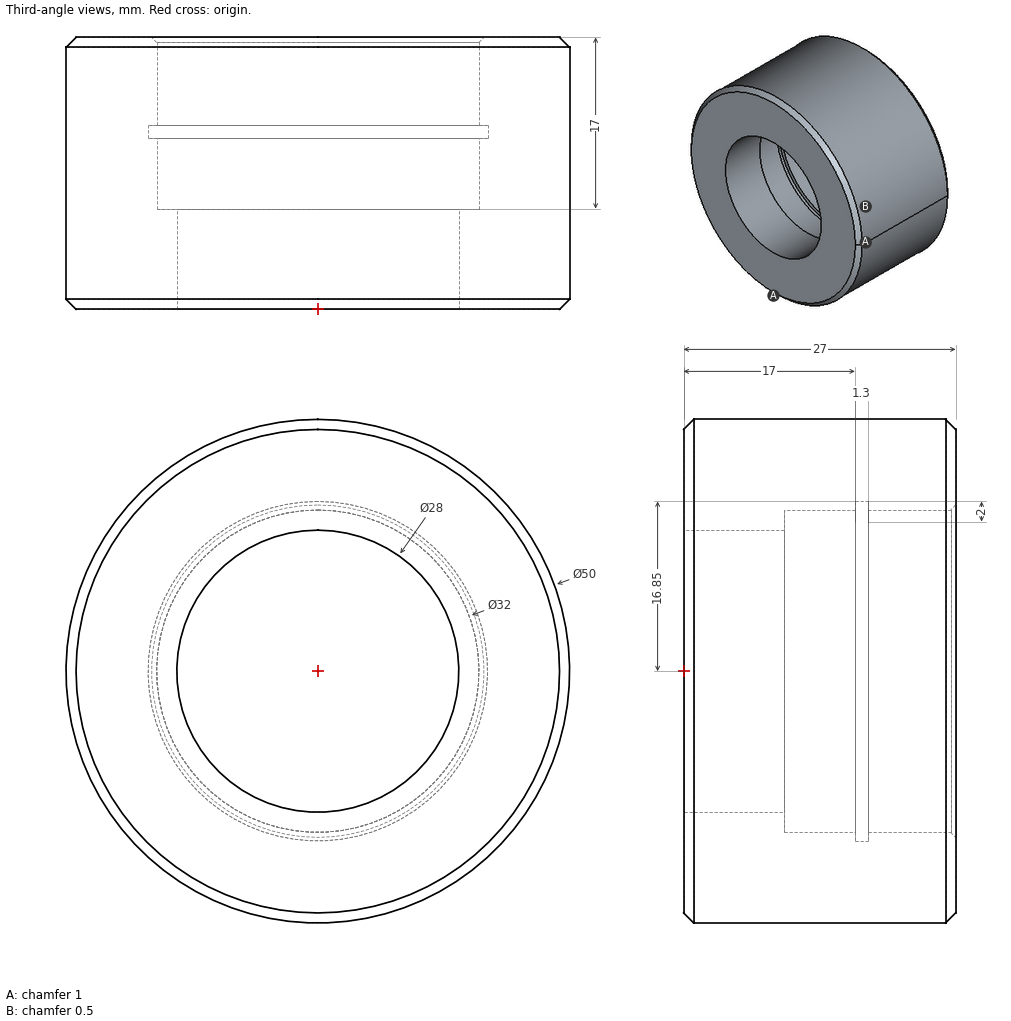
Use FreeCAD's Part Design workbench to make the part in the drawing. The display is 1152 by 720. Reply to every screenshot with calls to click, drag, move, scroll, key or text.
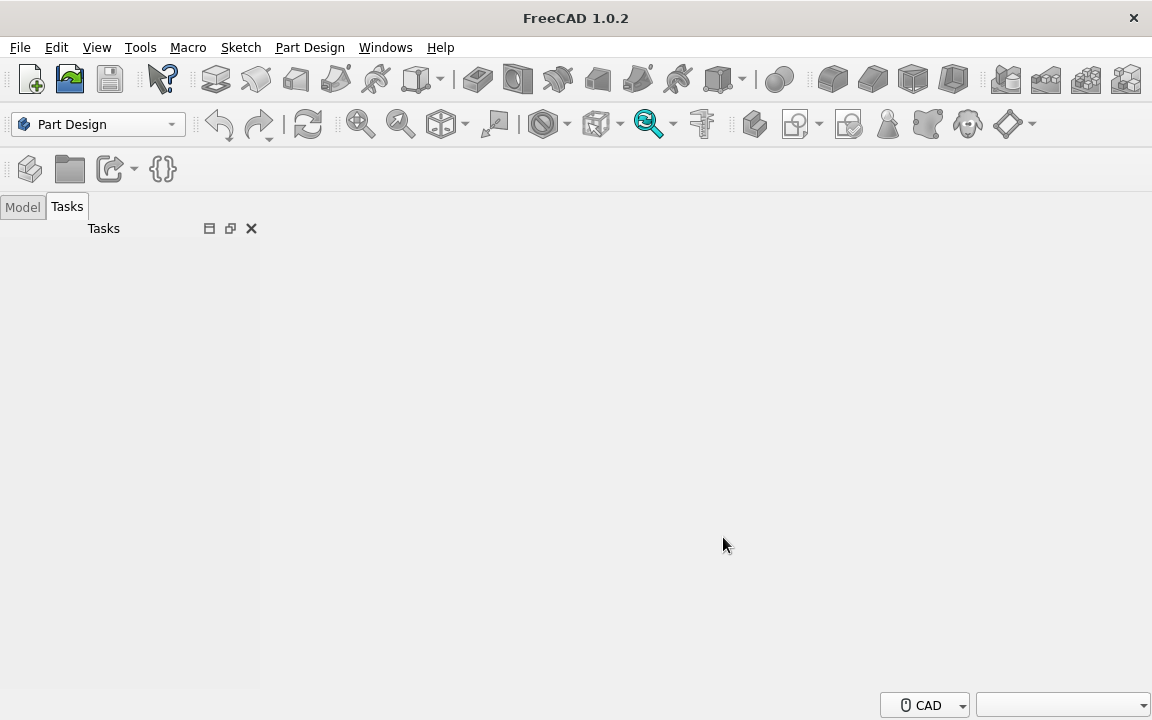
click(30, 80)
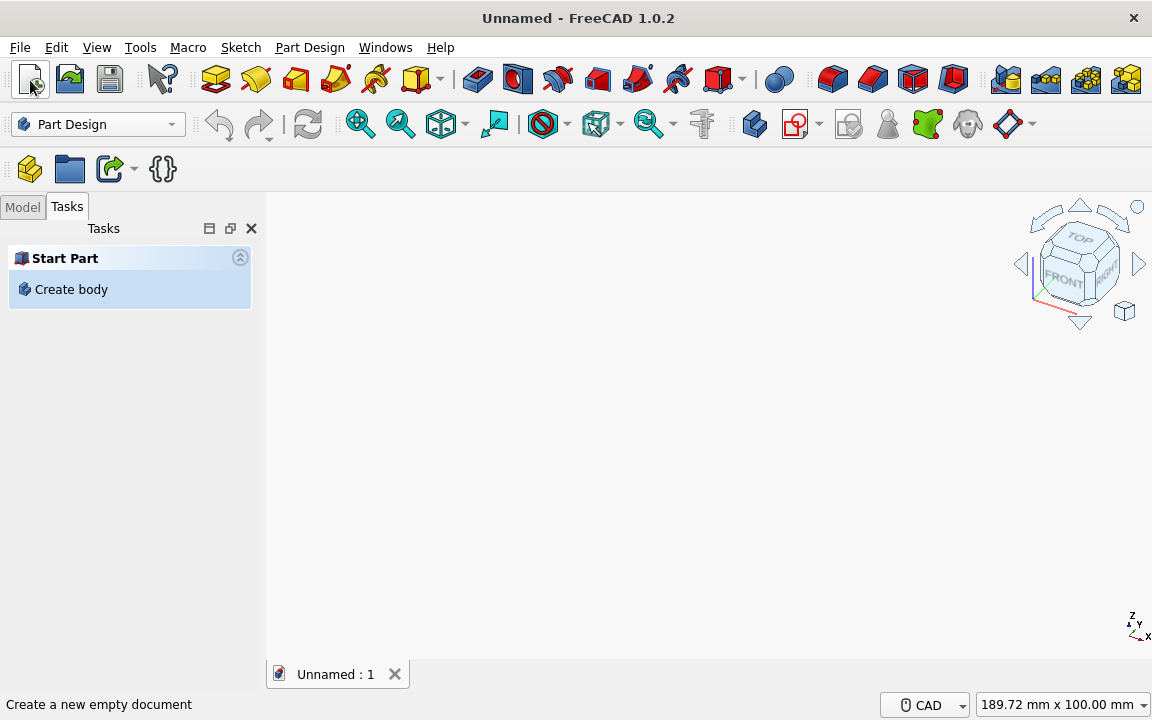
click(796, 124)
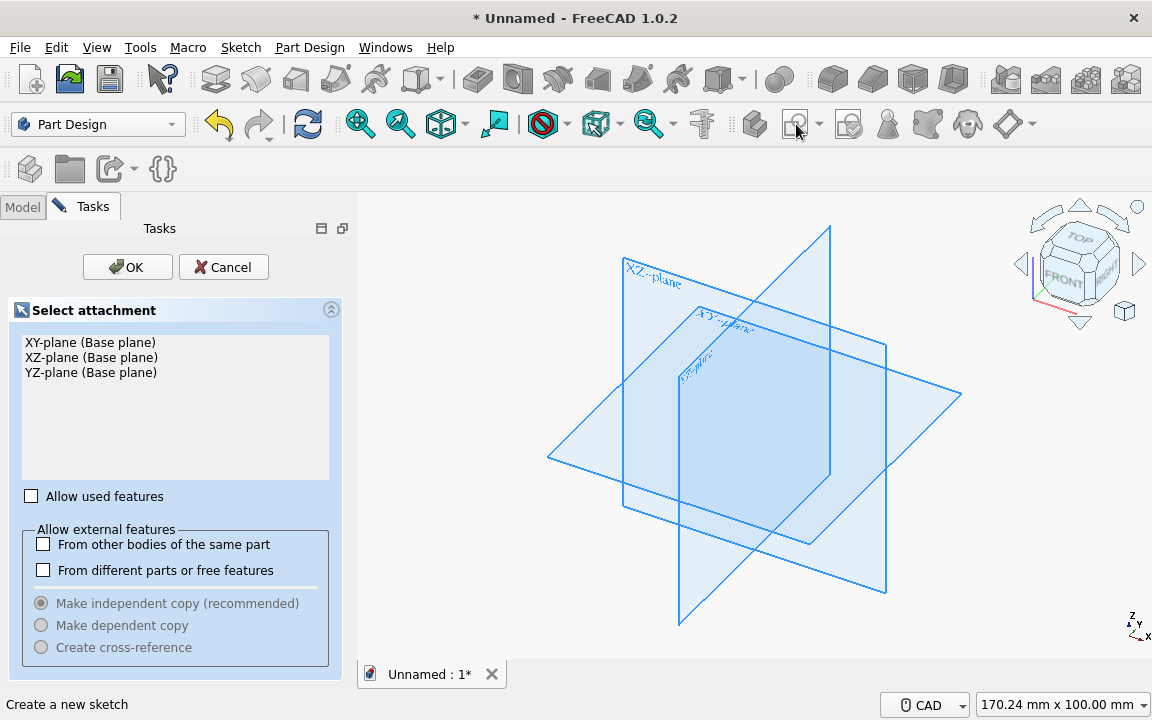
click(82, 358)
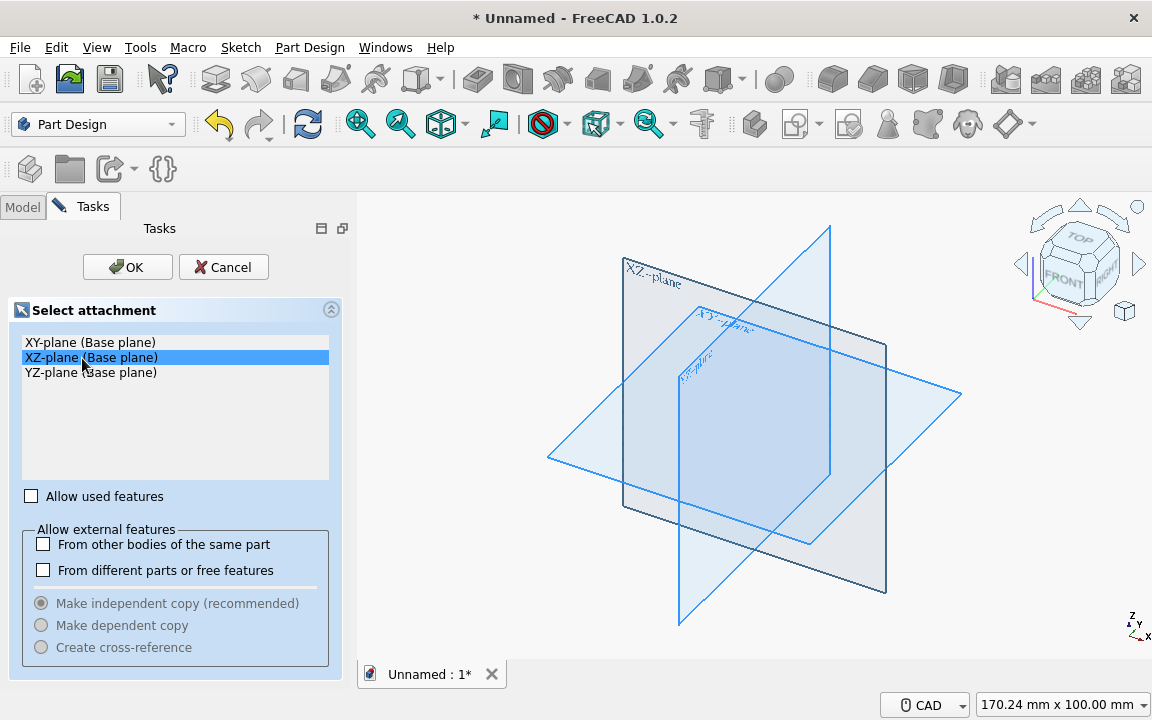
click(128, 267)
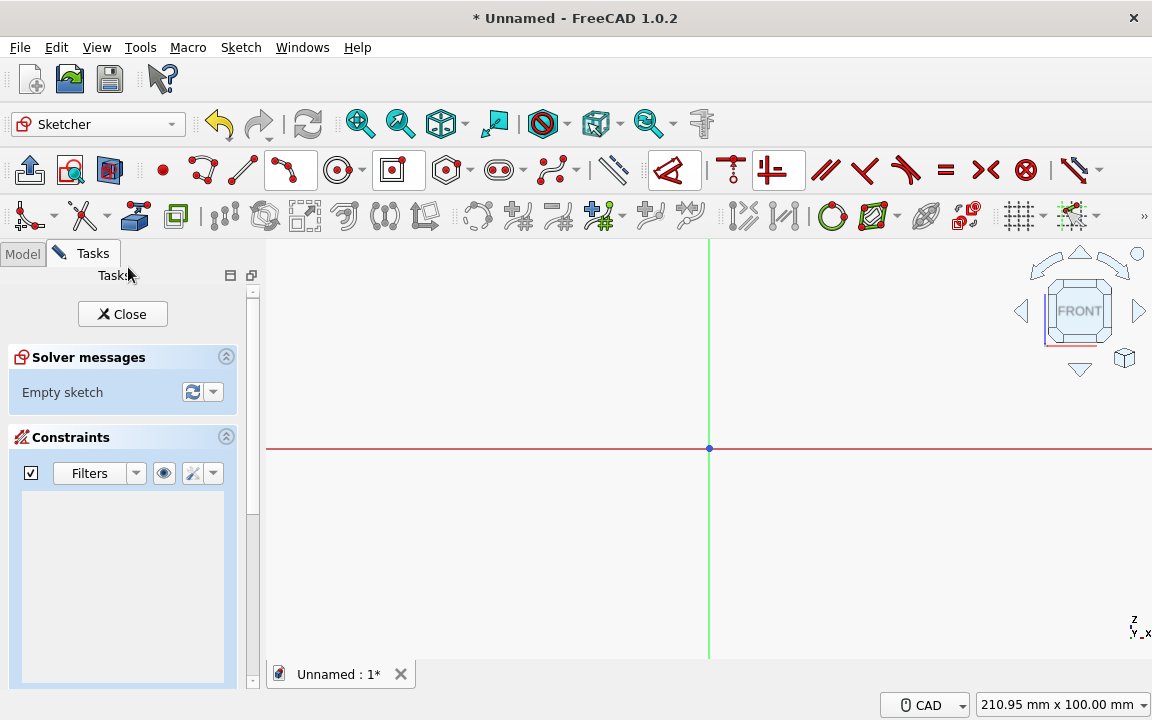
click(338, 170)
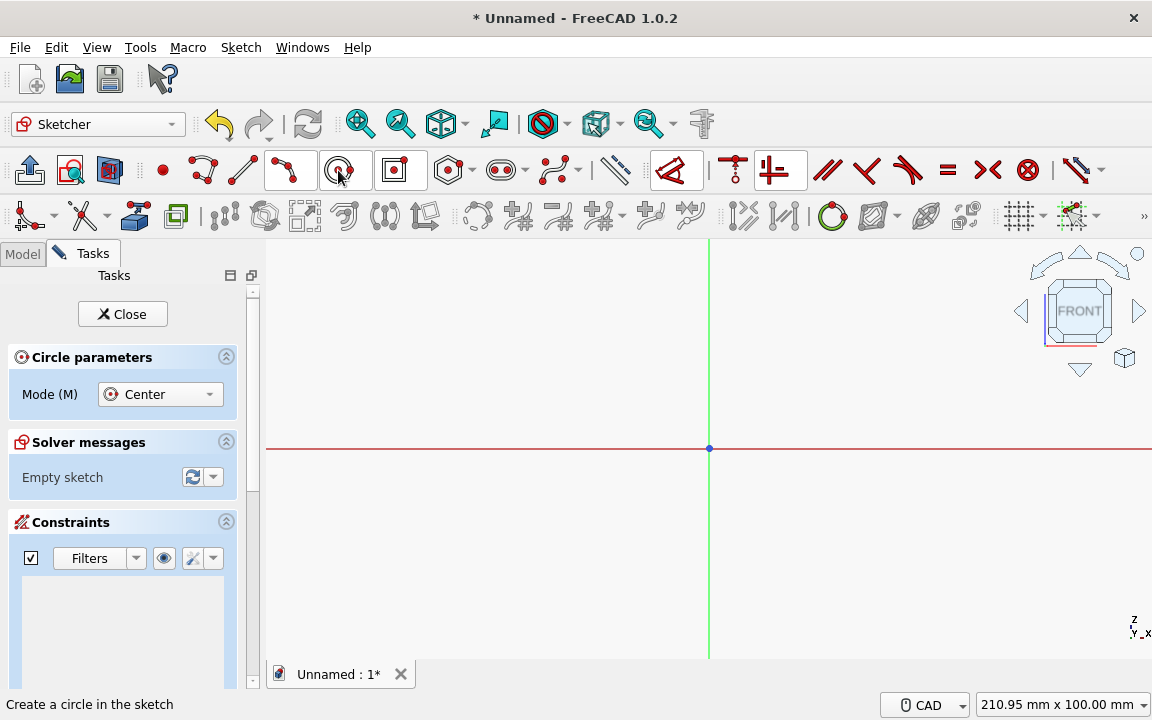
click(709, 449)
move(783, 375)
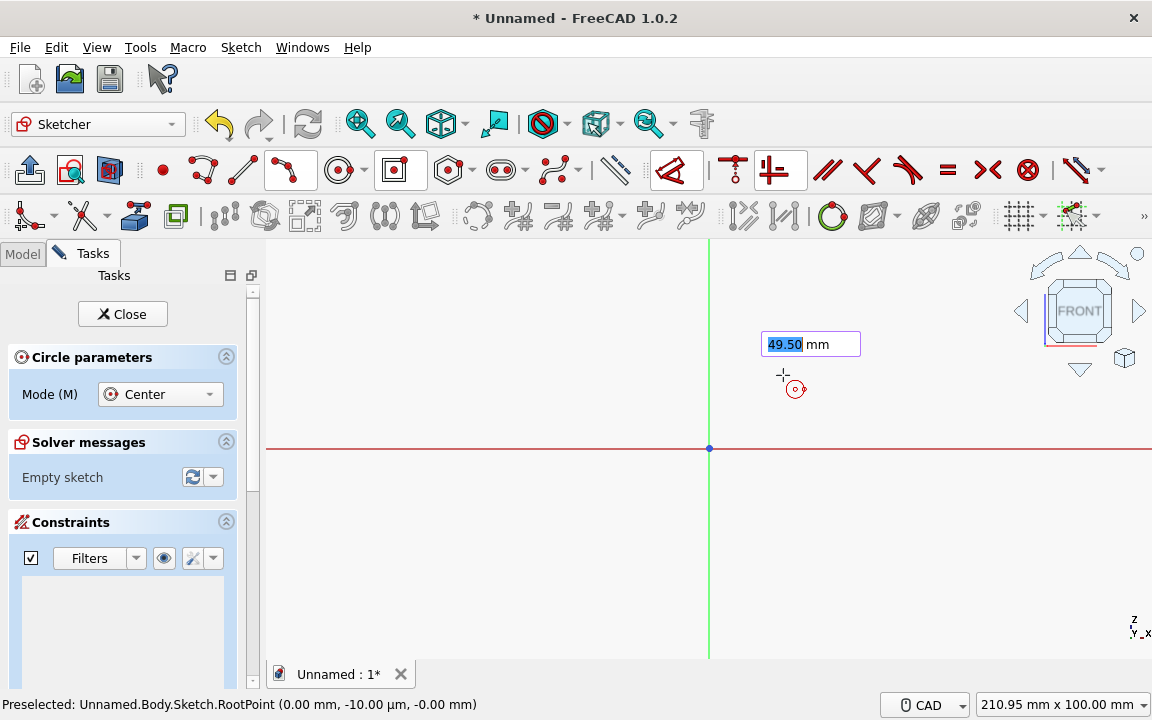
text(50)
key(Return)
key(Escape)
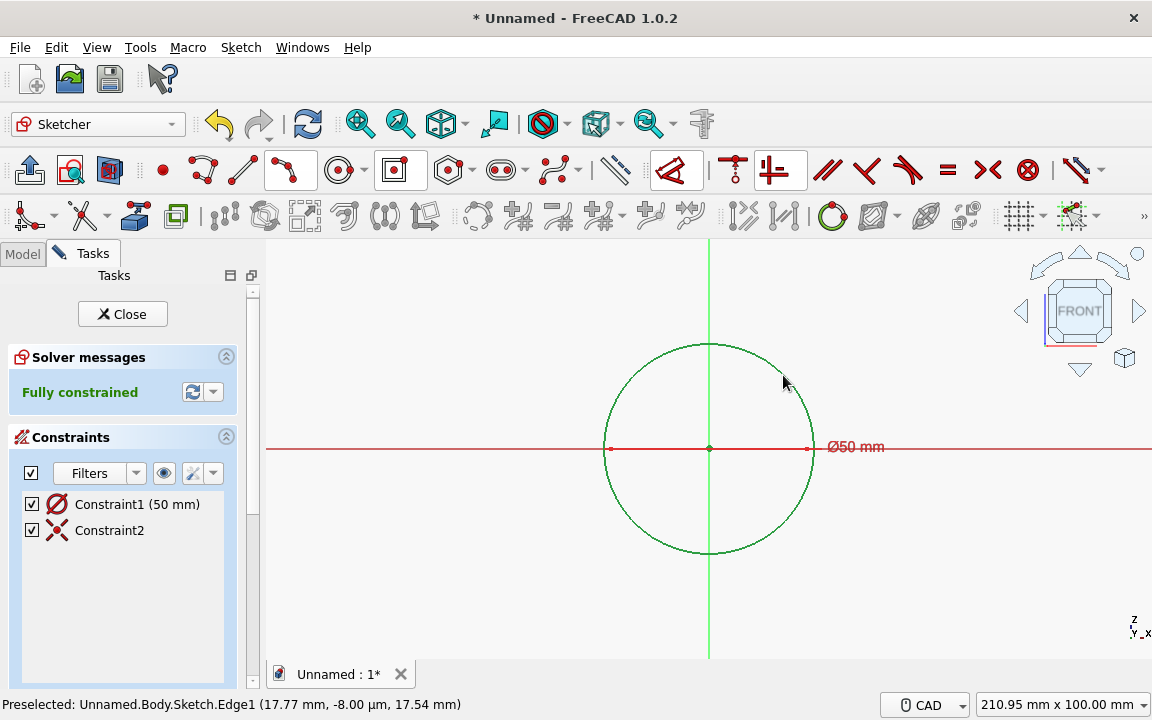
click(123, 314)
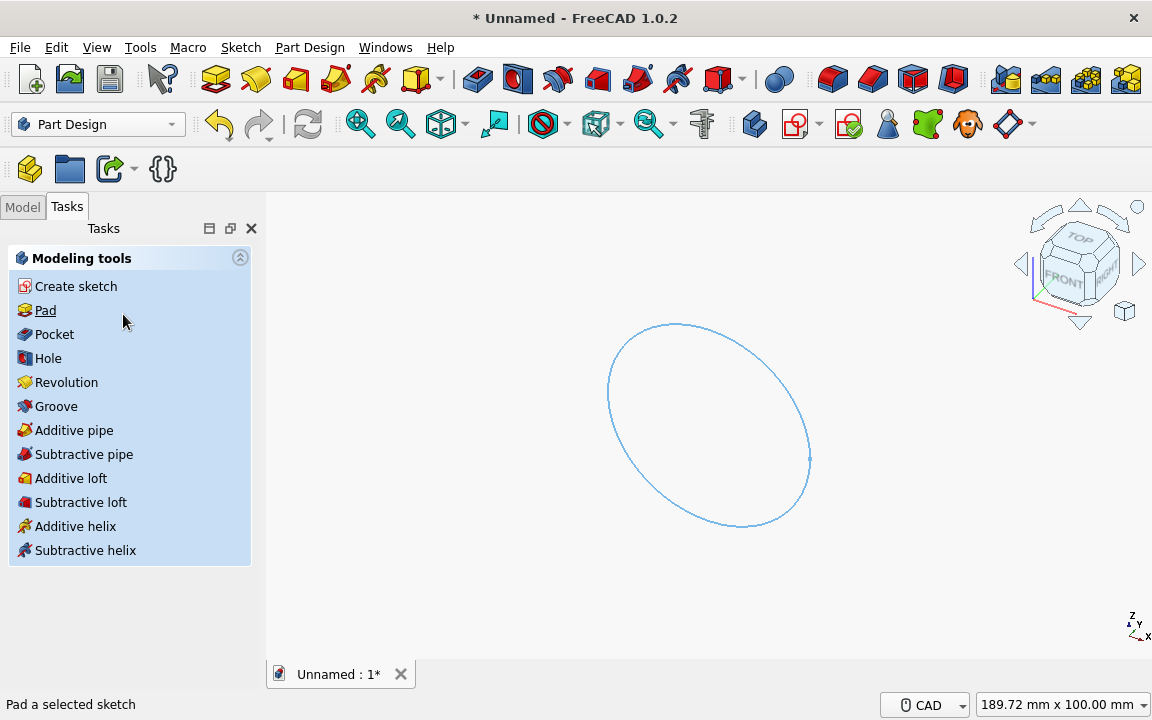
click(216, 80)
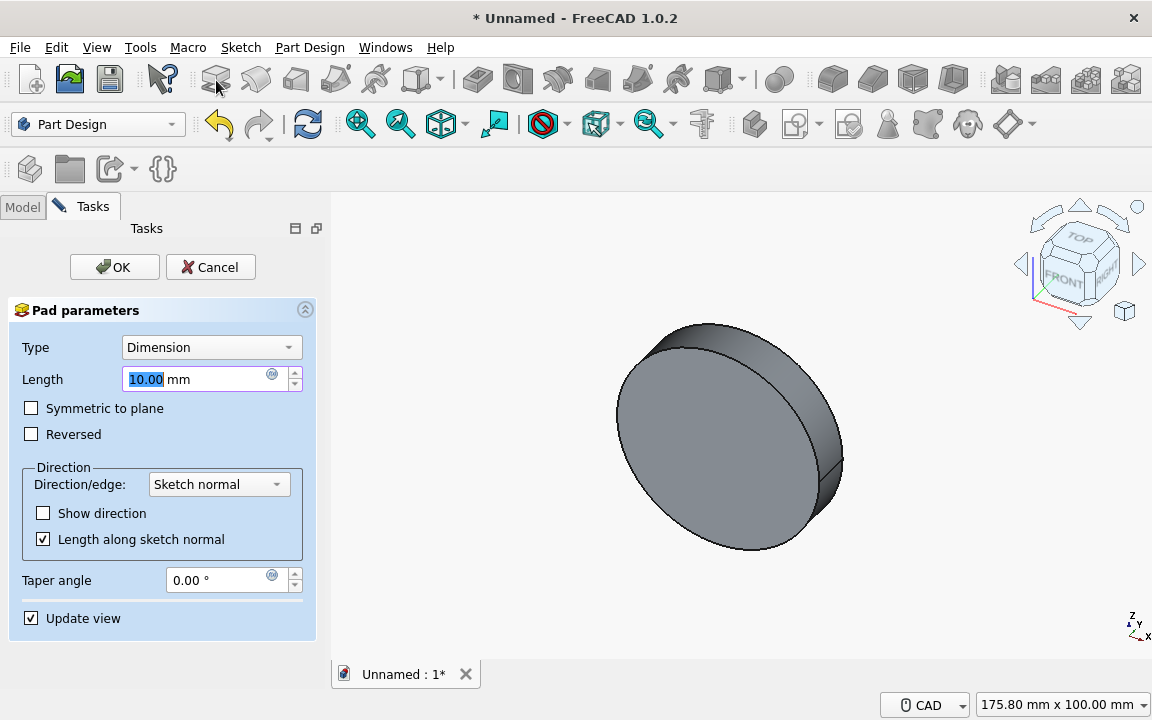
text(27)
key(Tab)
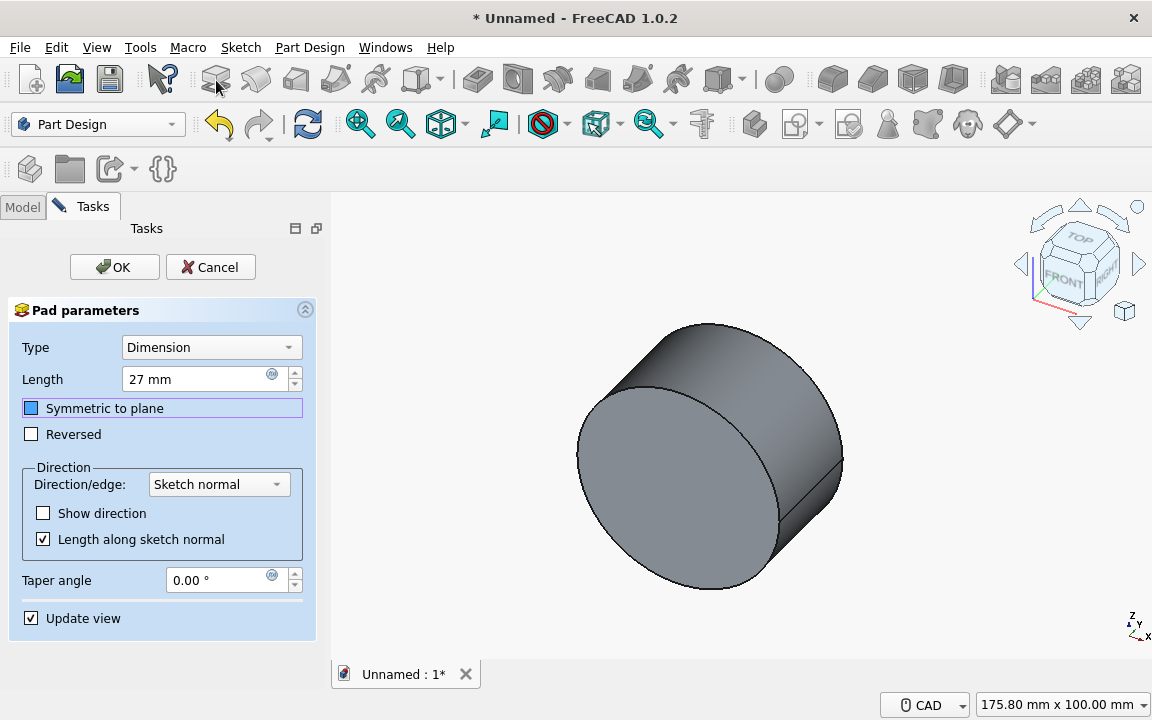
click(30, 434)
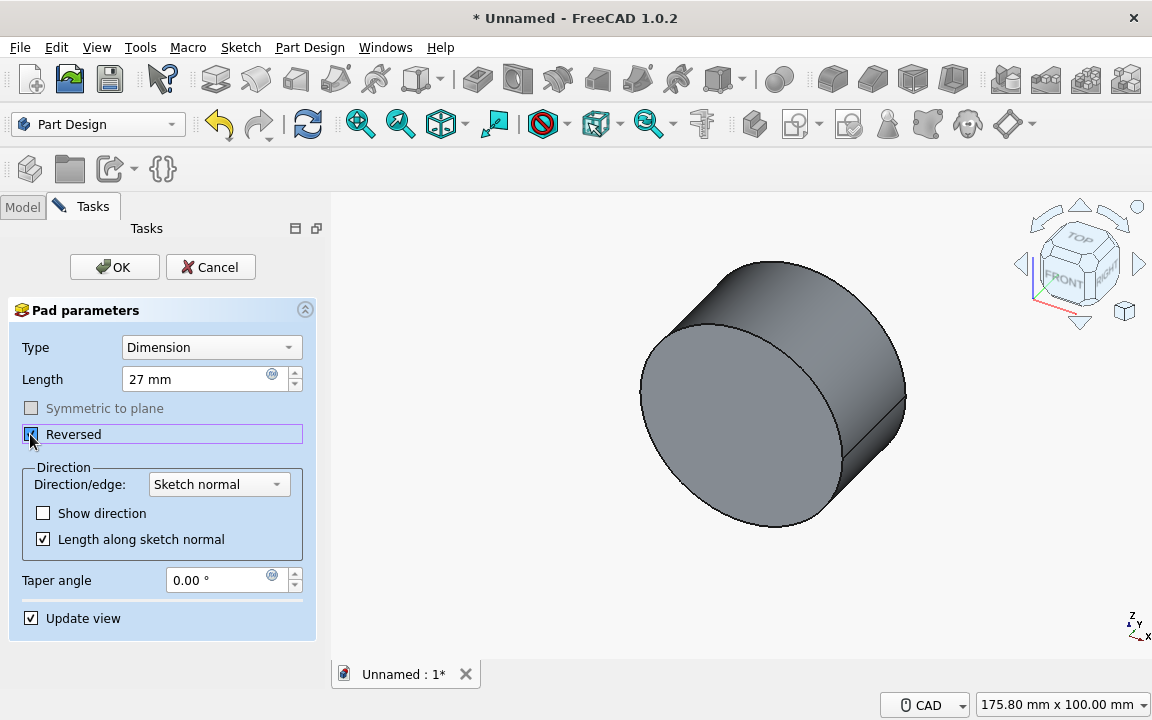
click(115, 267)